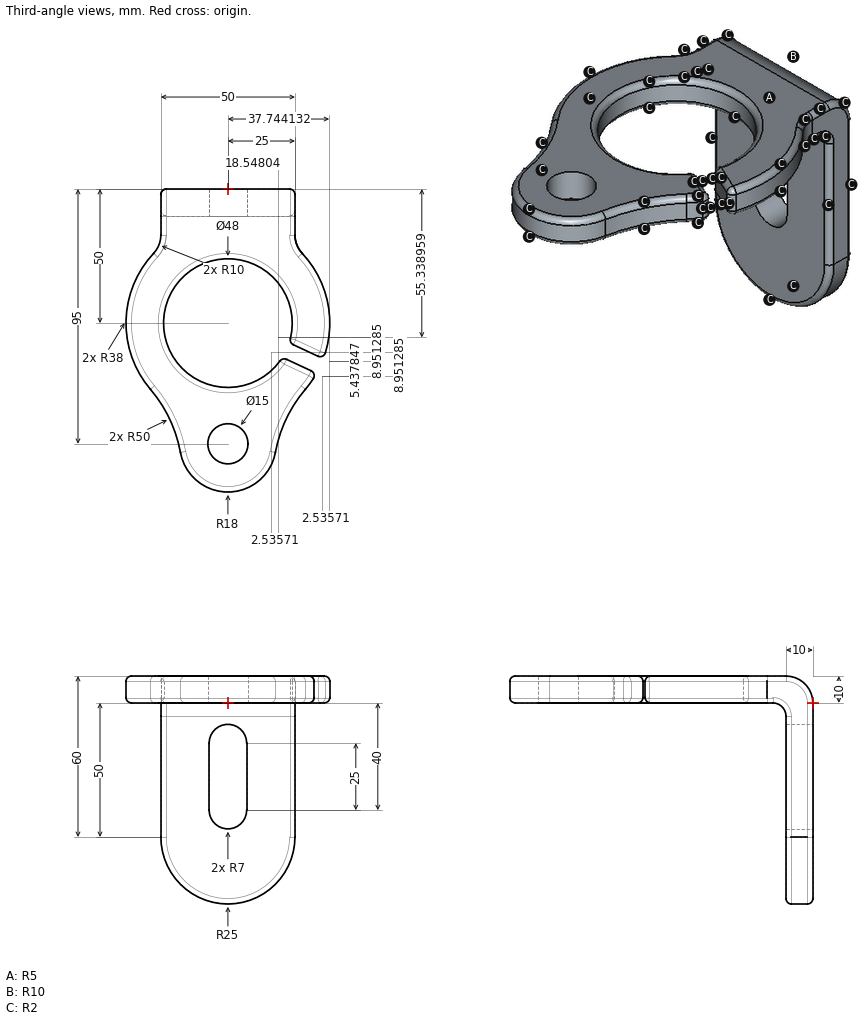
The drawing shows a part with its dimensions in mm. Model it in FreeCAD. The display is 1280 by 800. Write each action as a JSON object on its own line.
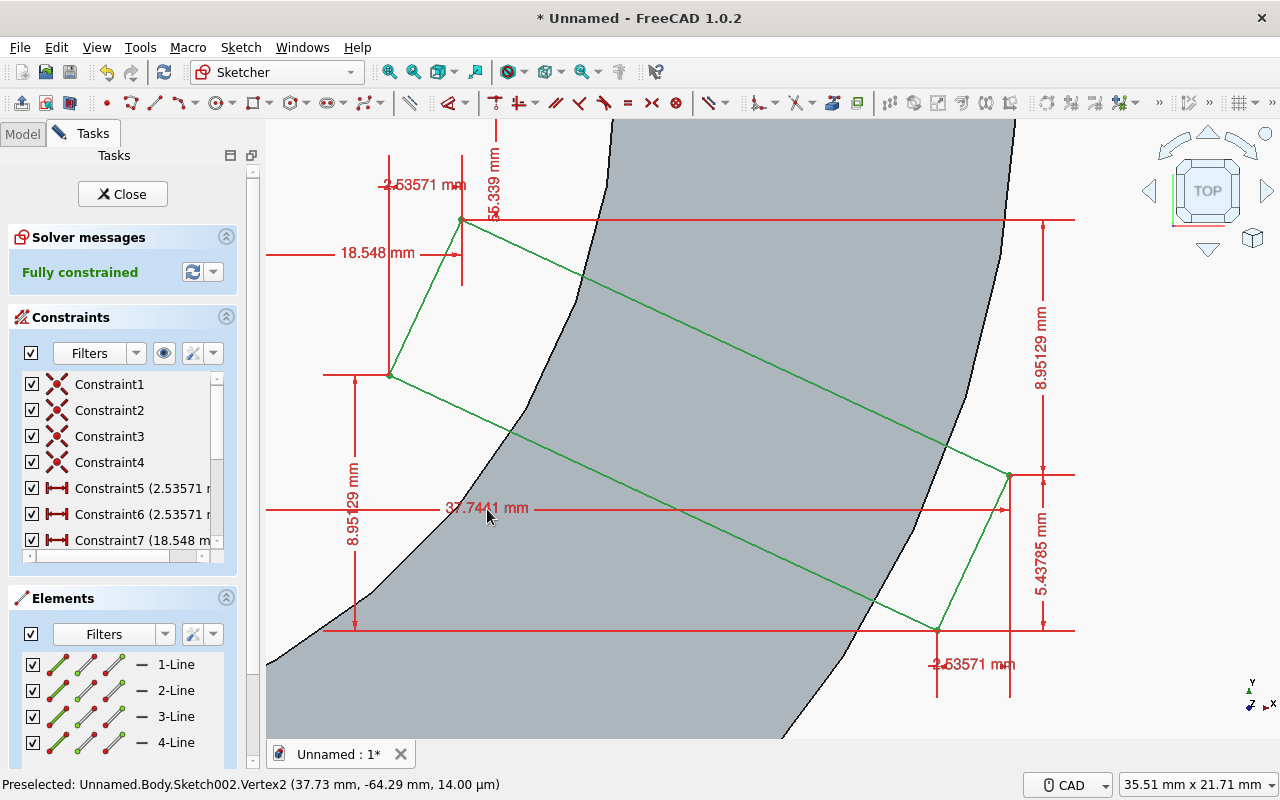
{"action": "left_click", "coordinate": [123, 194]}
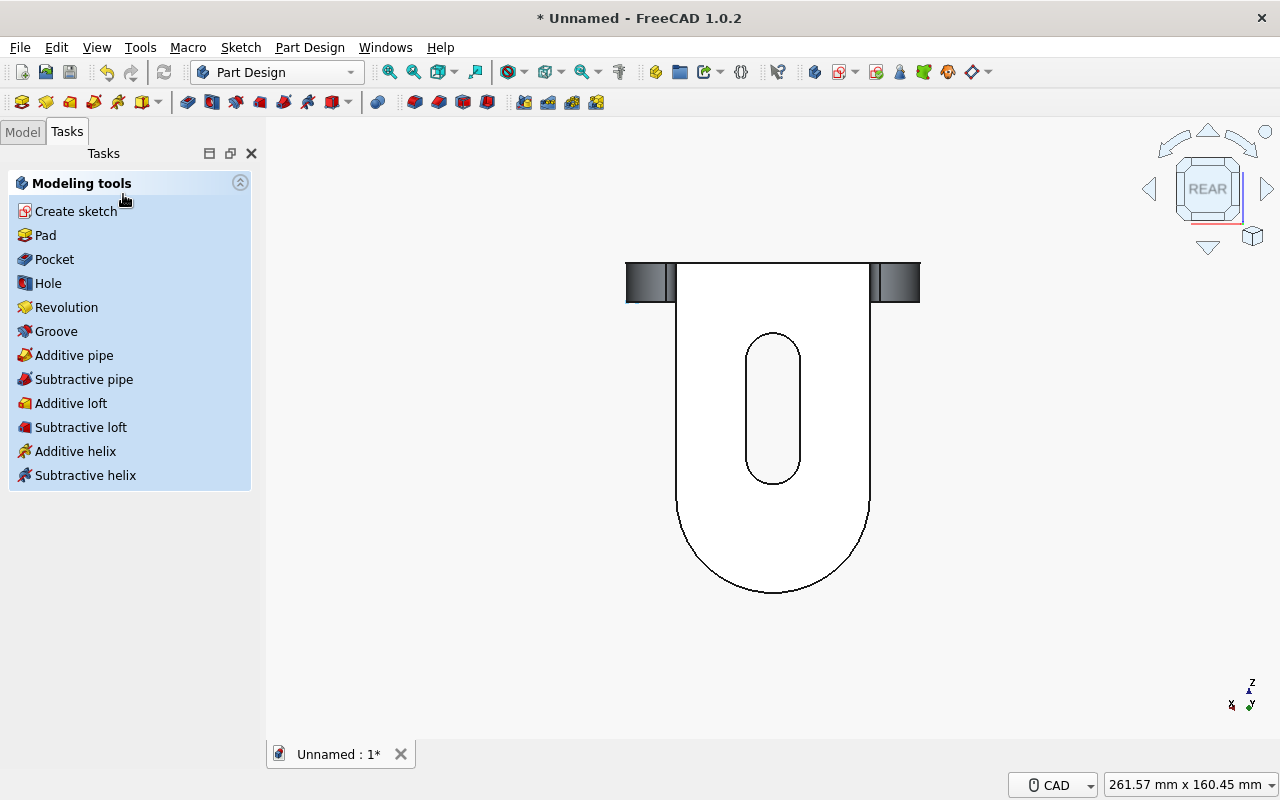
{"action": "left_click", "coordinate": [188, 102]}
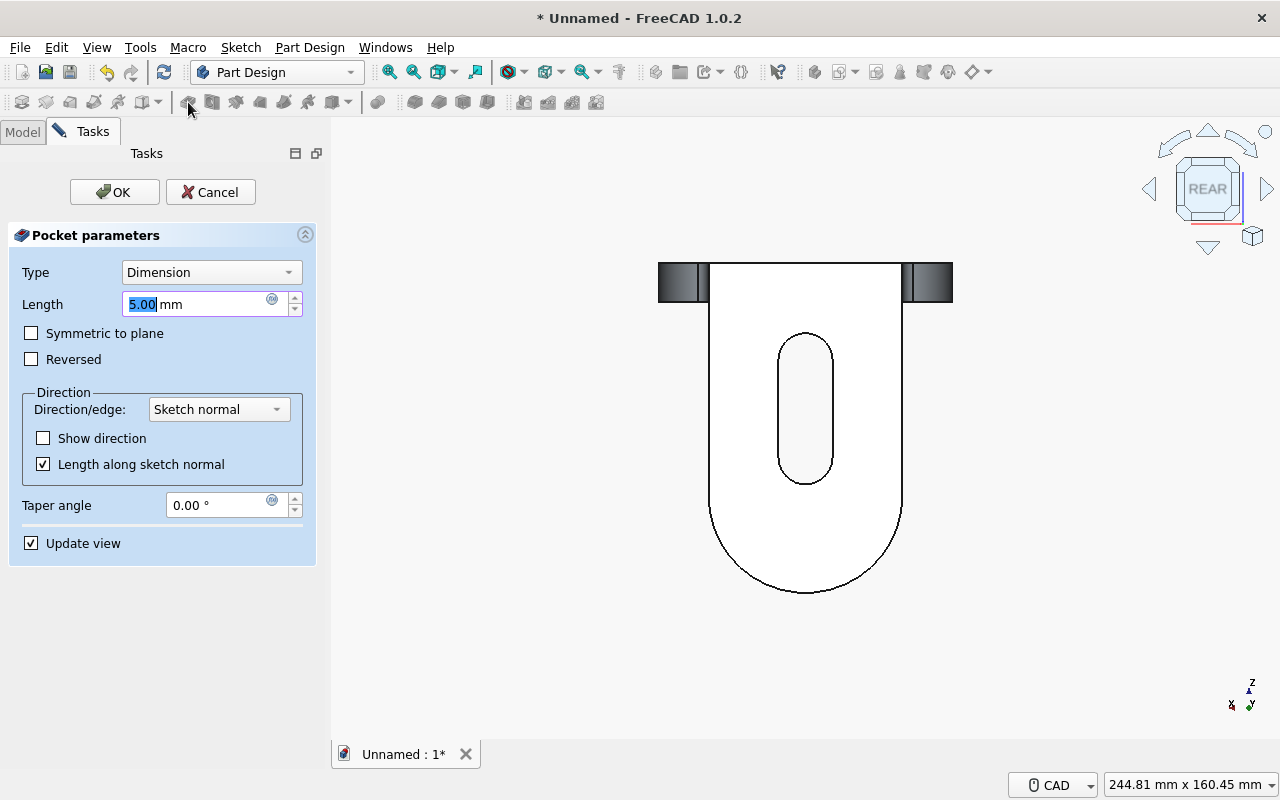
{"action": "left_click", "coordinate": [212, 272]}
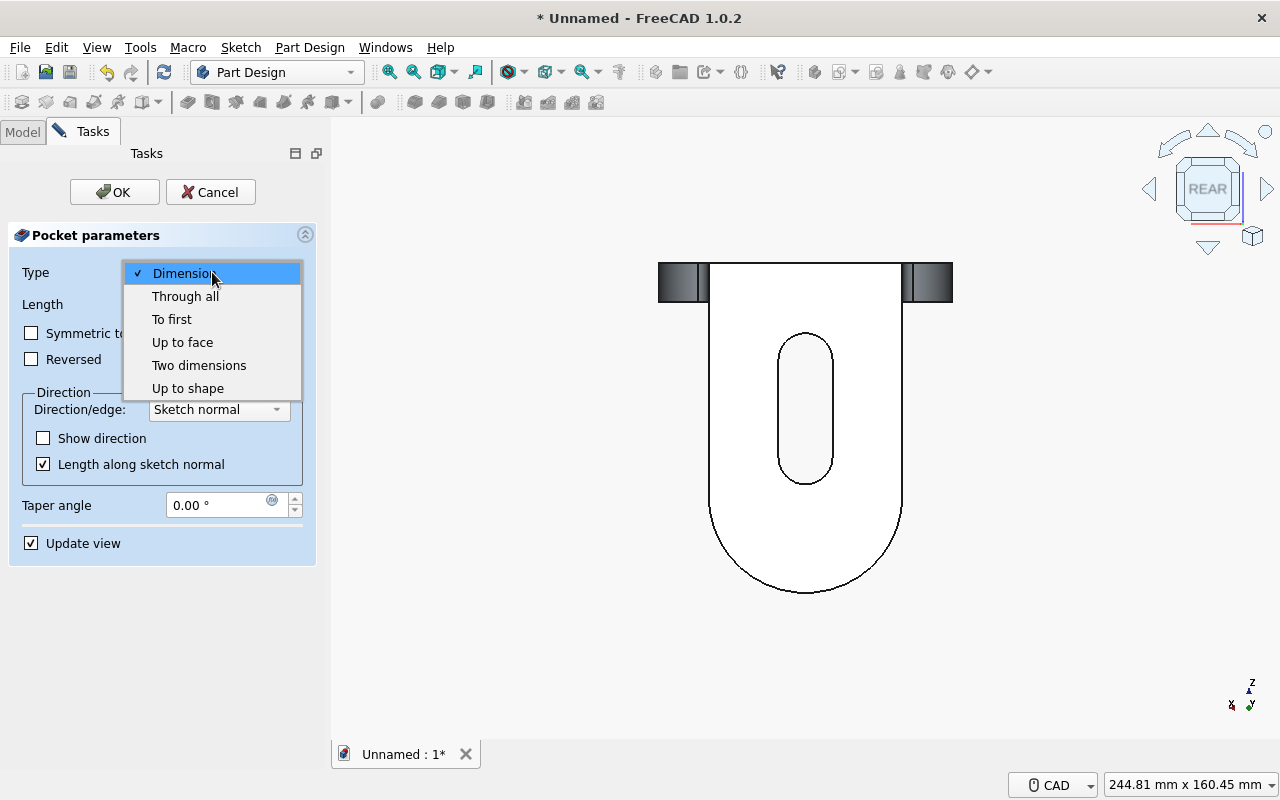
{"action": "left_click", "coordinate": [212, 296]}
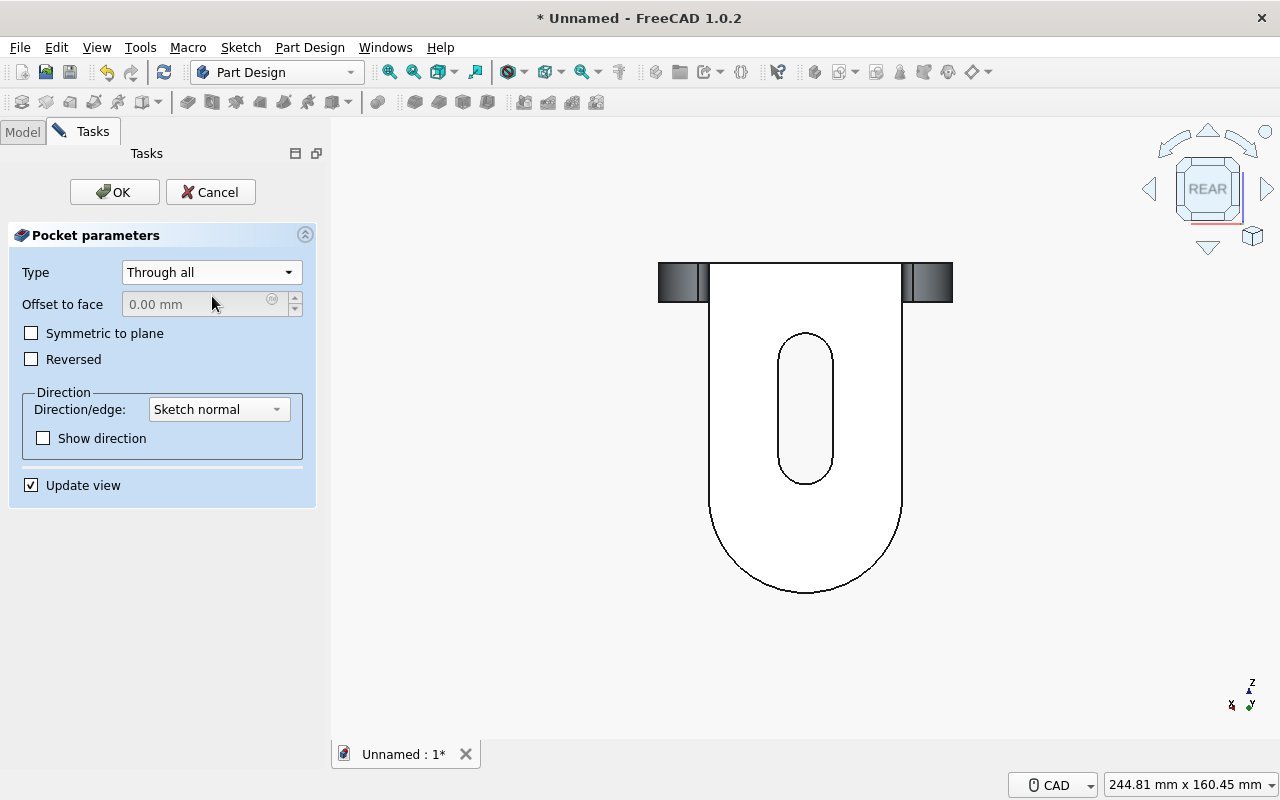
{"action": "left_click", "coordinate": [30, 359]}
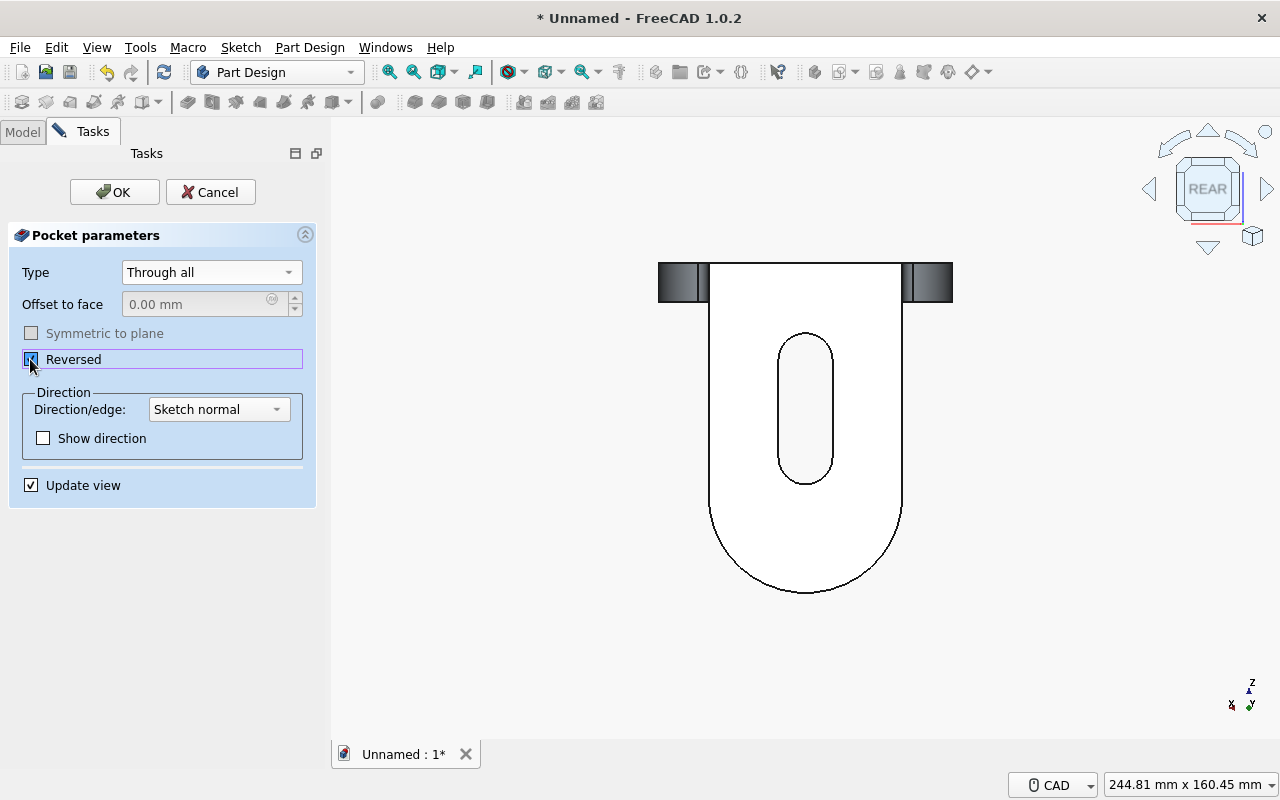
{"action": "left_click", "coordinate": [115, 192]}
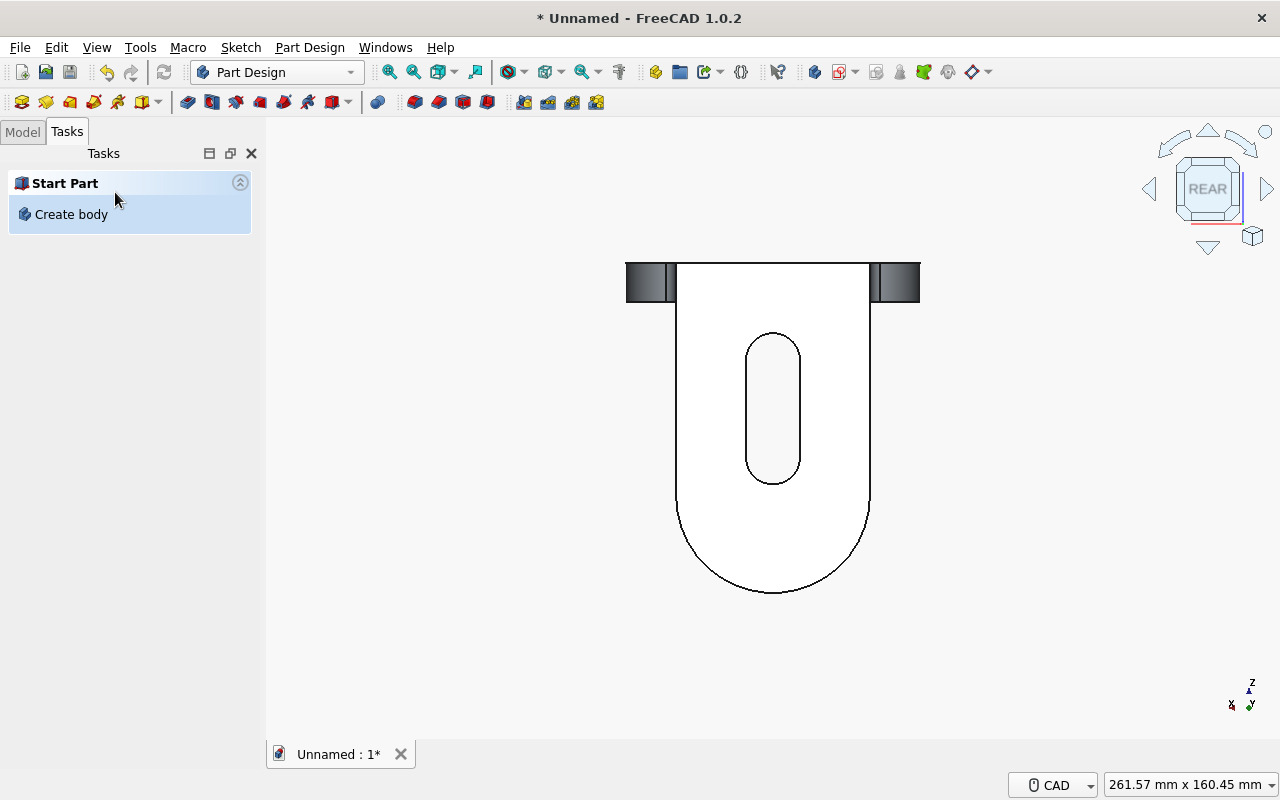
{"action": "key", "text": "0"}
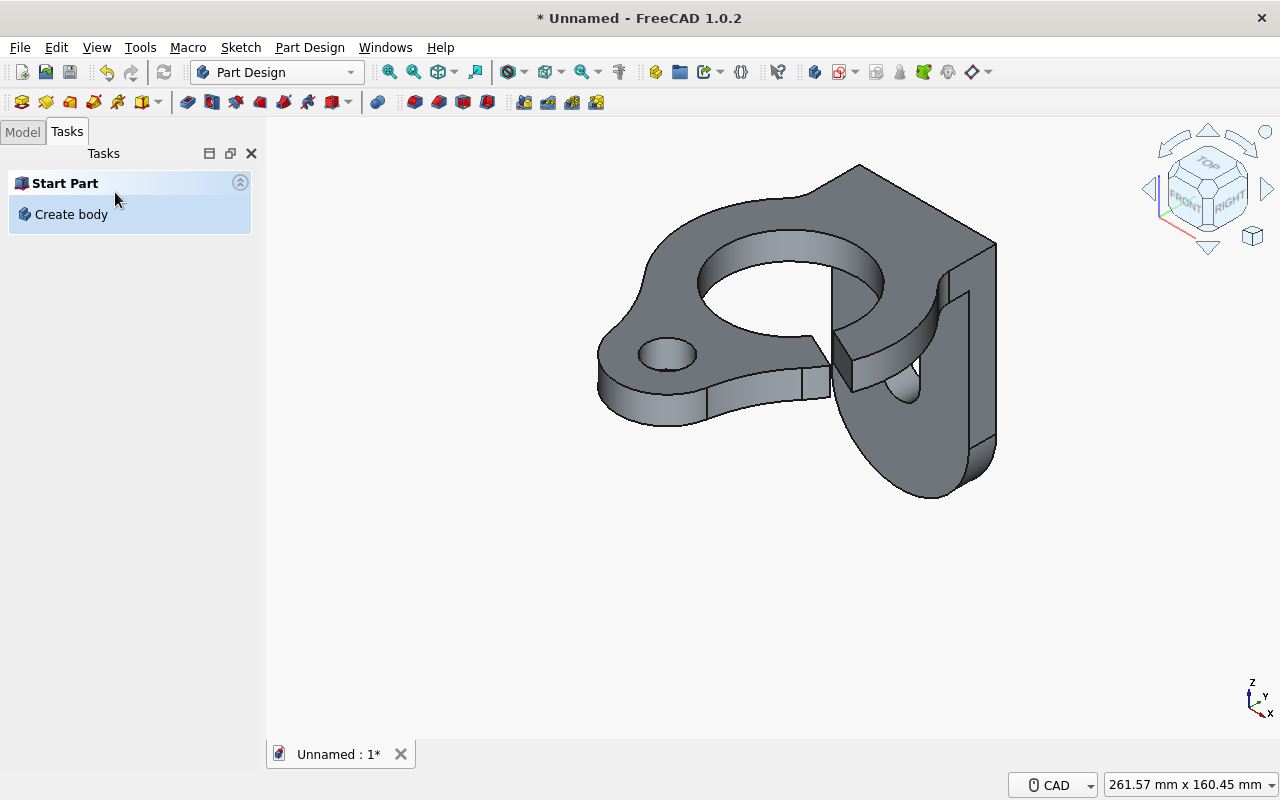
{"action": "key", "text": "2"}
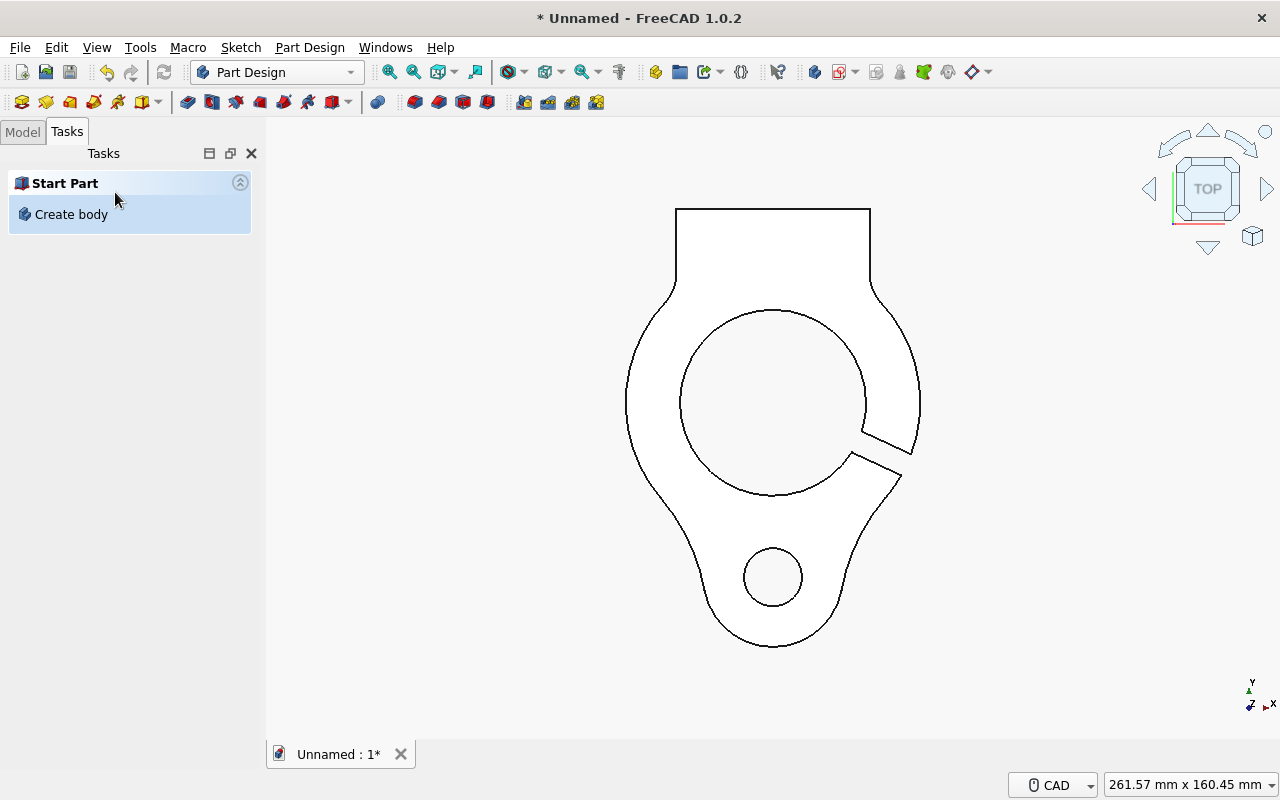
{"action": "key", "text": "1"}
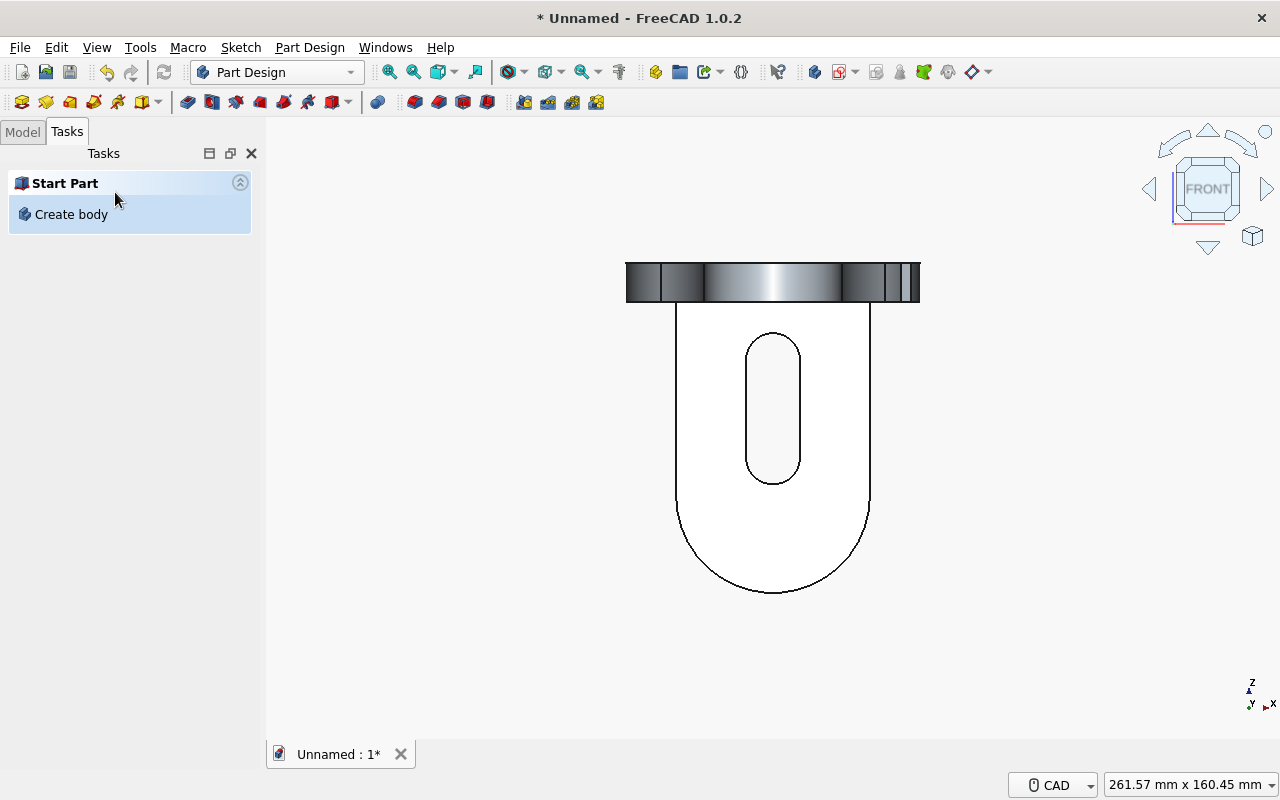
{"action": "key", "text": "3"}